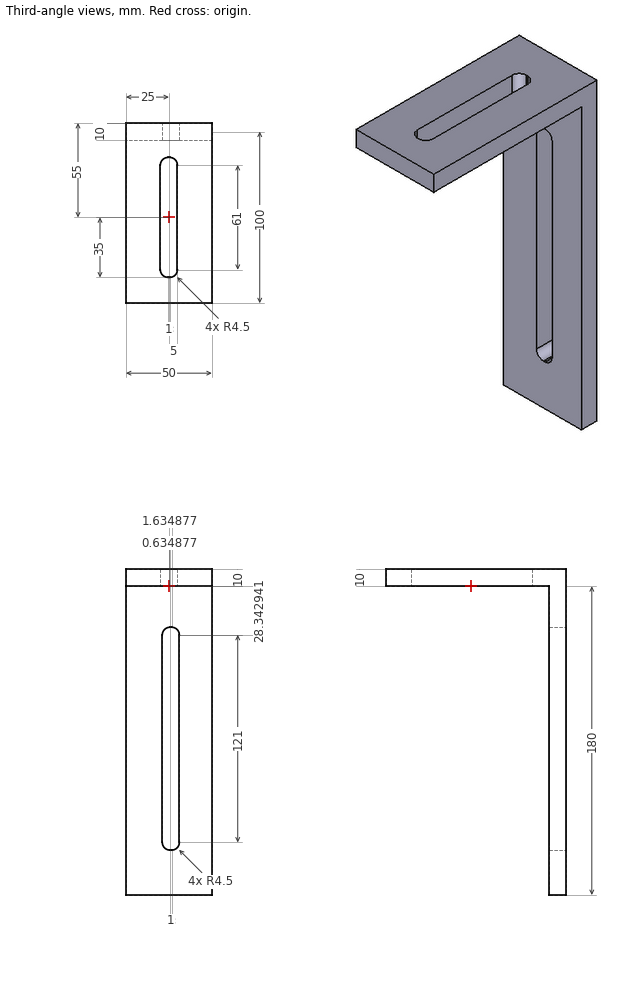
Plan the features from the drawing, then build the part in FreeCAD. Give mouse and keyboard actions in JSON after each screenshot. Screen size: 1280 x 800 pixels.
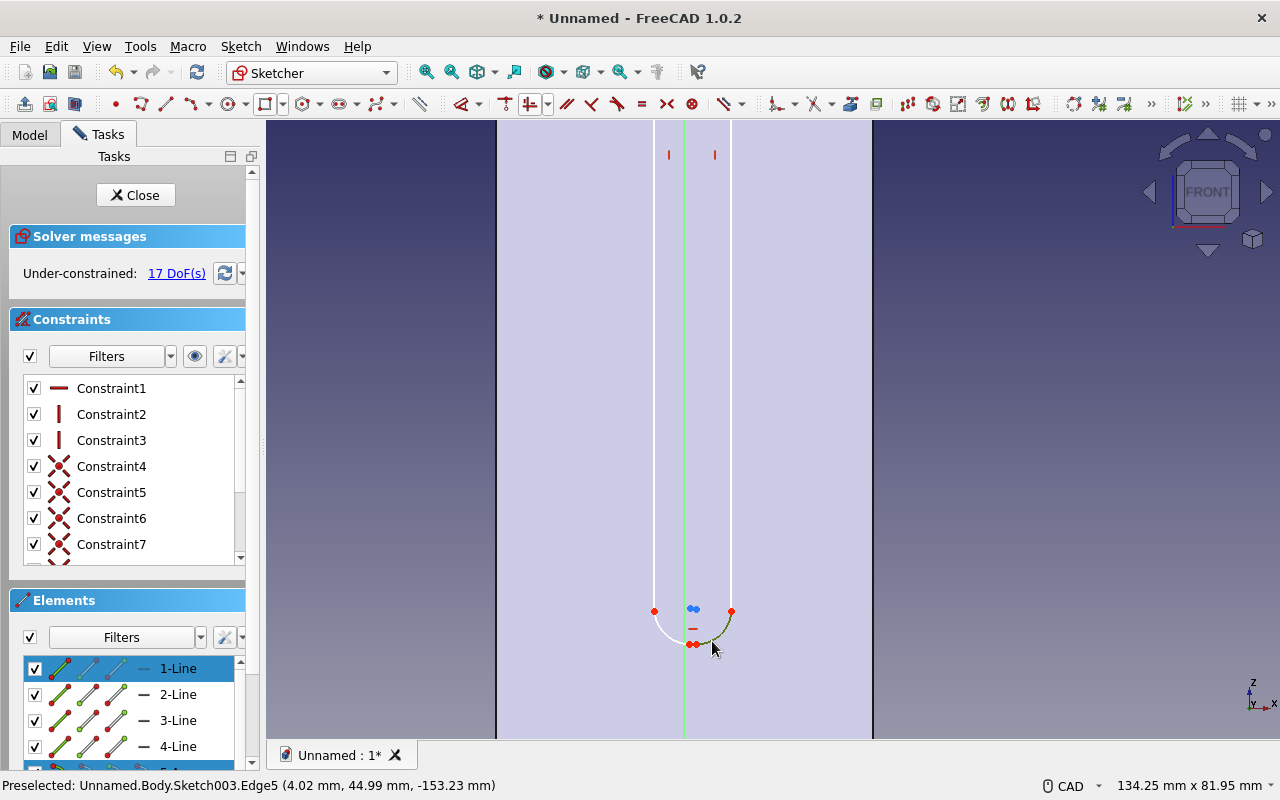
{"action": "left_click", "coordinate": [617, 104]}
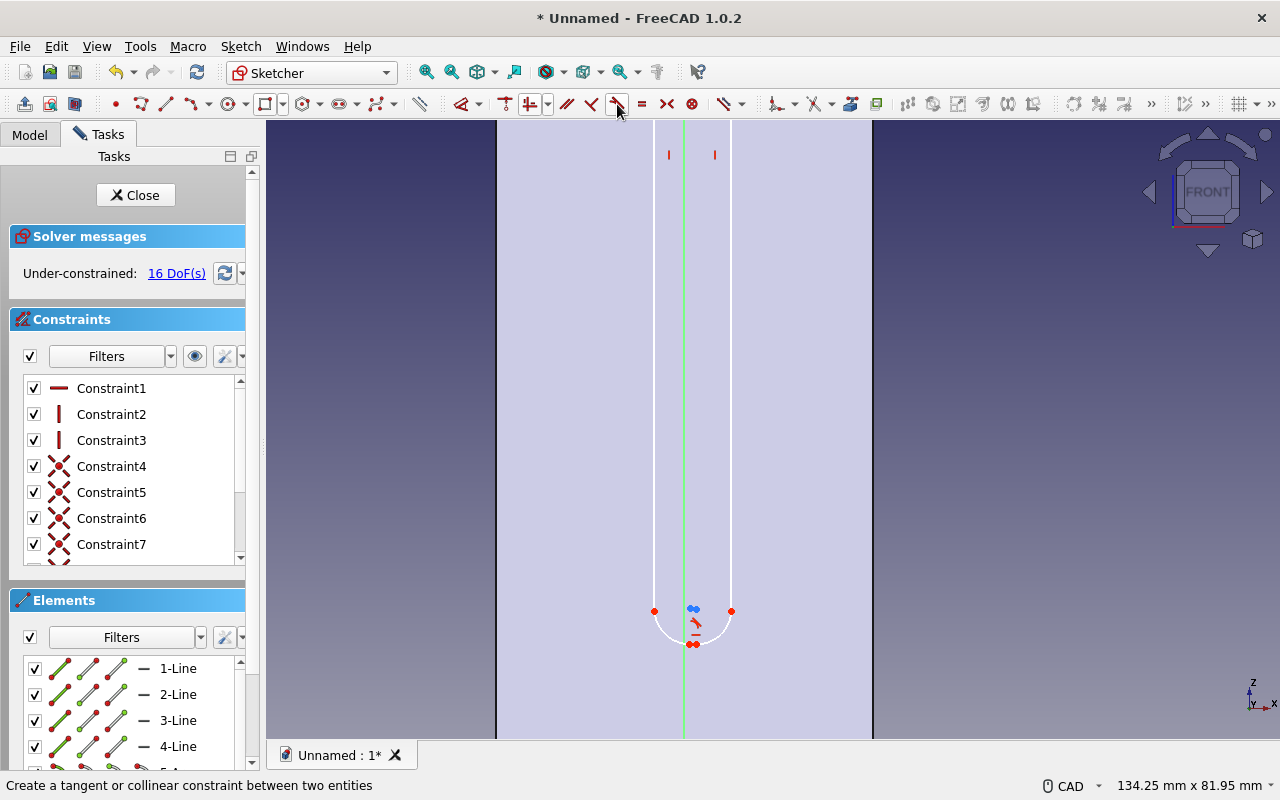
{"action": "scroll", "coordinate": [693, 644], "scroll_direction": "up", "scroll_amount": 7}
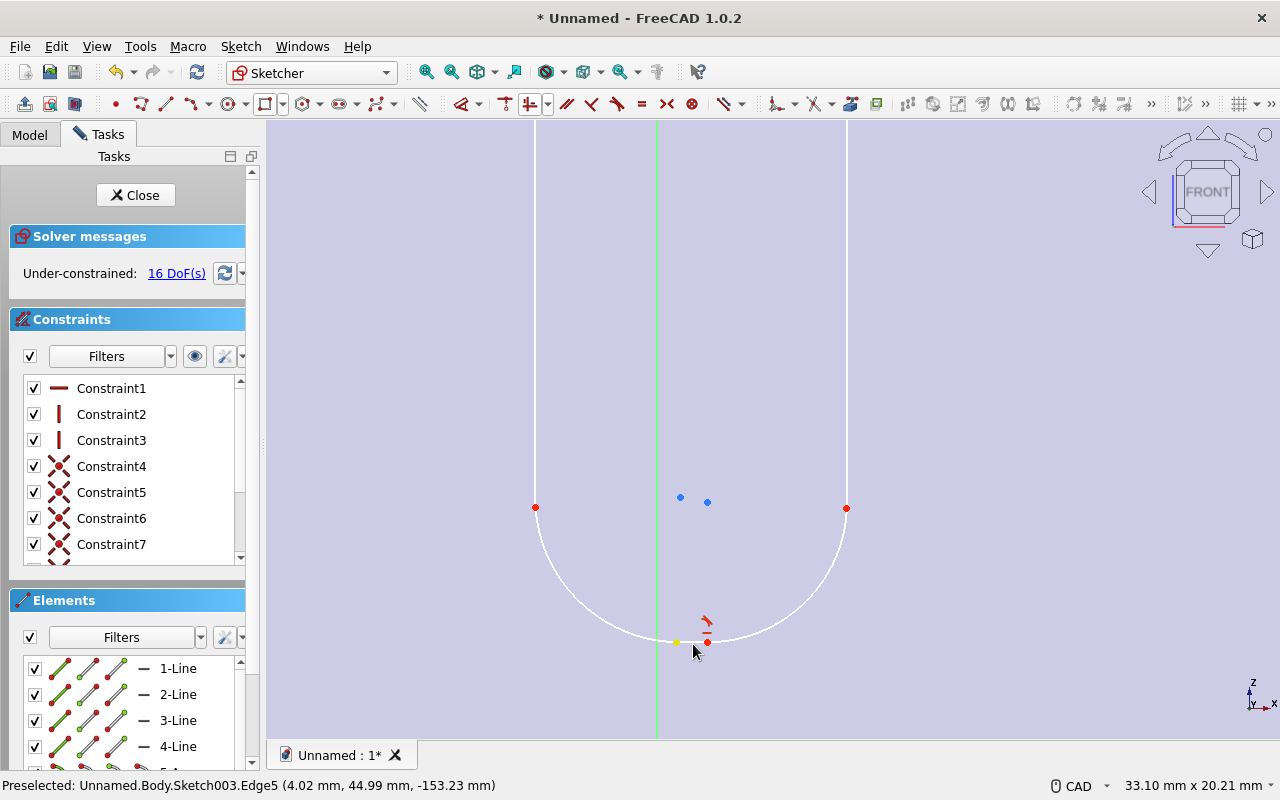
{"action": "left_click", "coordinate": [692, 642]}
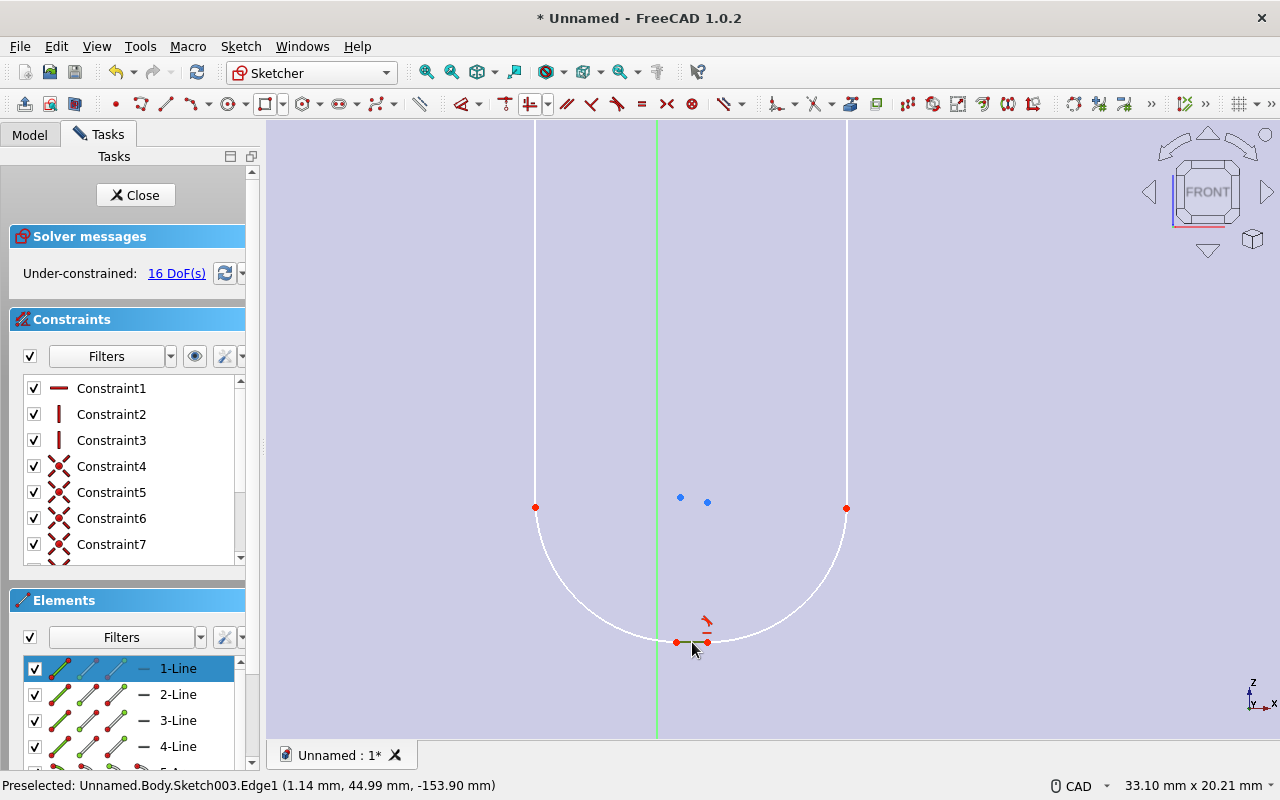
{"action": "scroll", "coordinate": [706, 644], "scroll_direction": "down", "scroll_amount": 12}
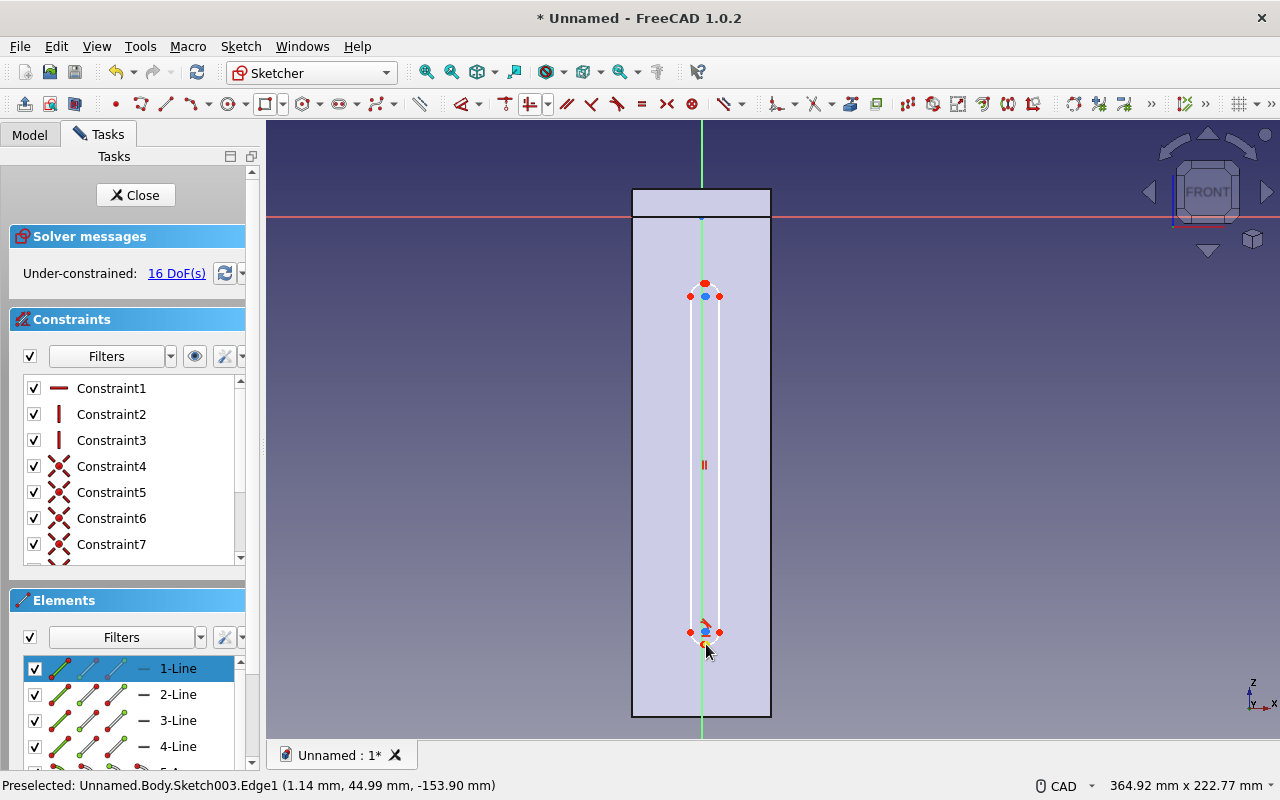
{"action": "scroll", "coordinate": [693, 638], "scroll_direction": "up", "scroll_amount": 5}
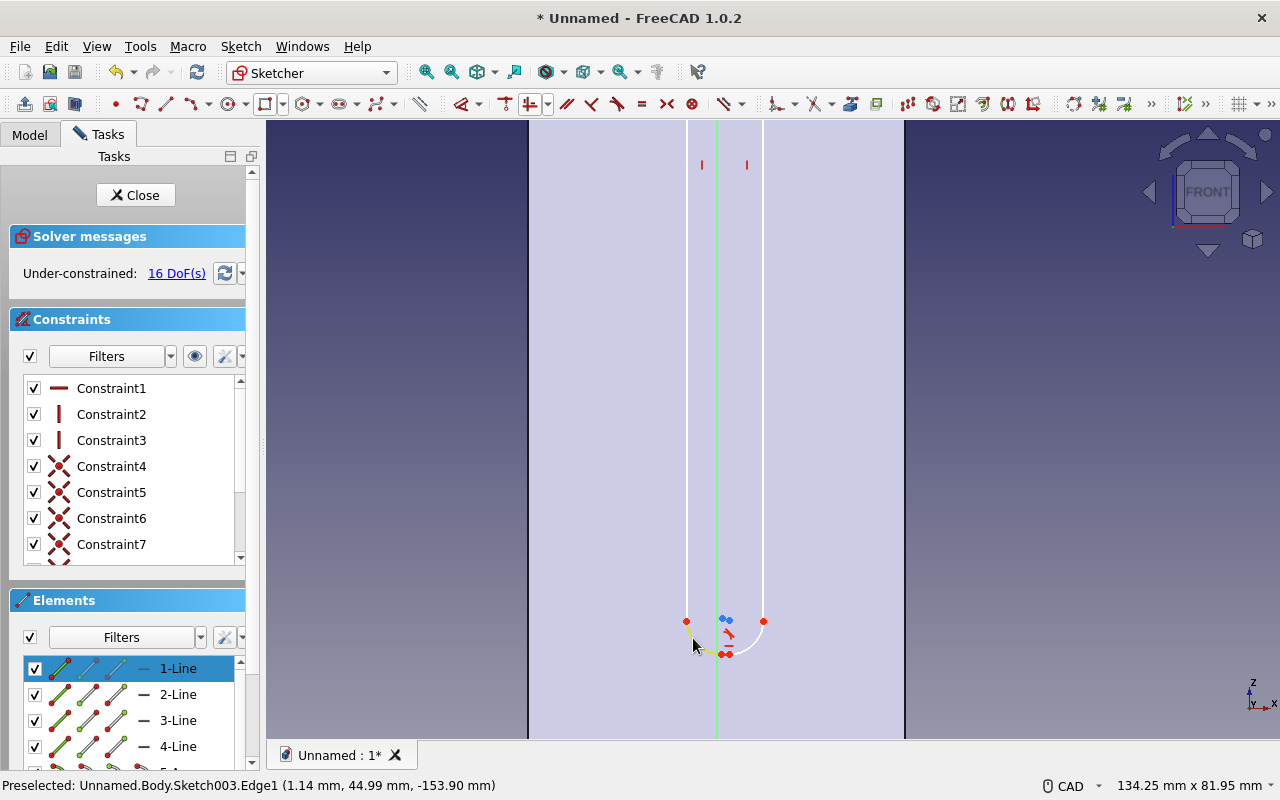
{"action": "left_click", "coordinate": [691, 636]}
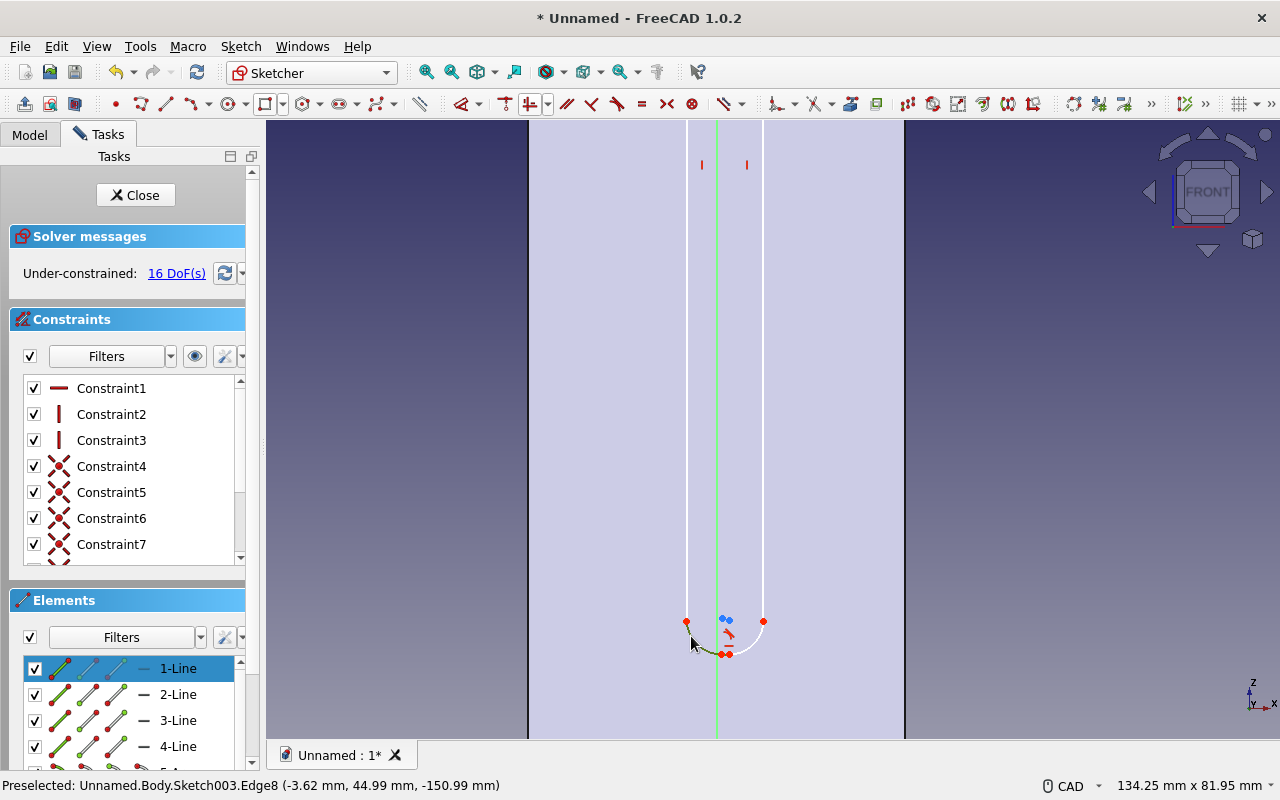
{"action": "left_click", "coordinate": [617, 104]}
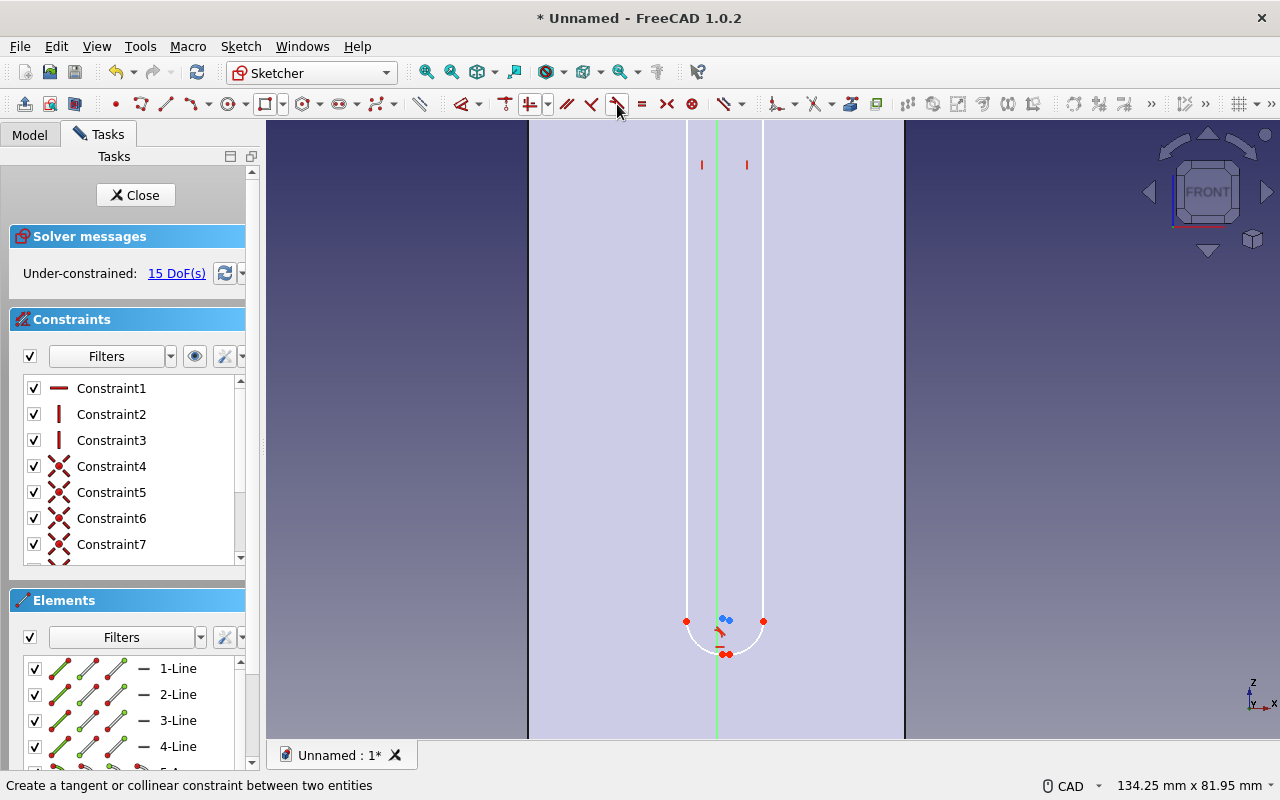
{"action": "left_click", "coordinate": [763, 348]}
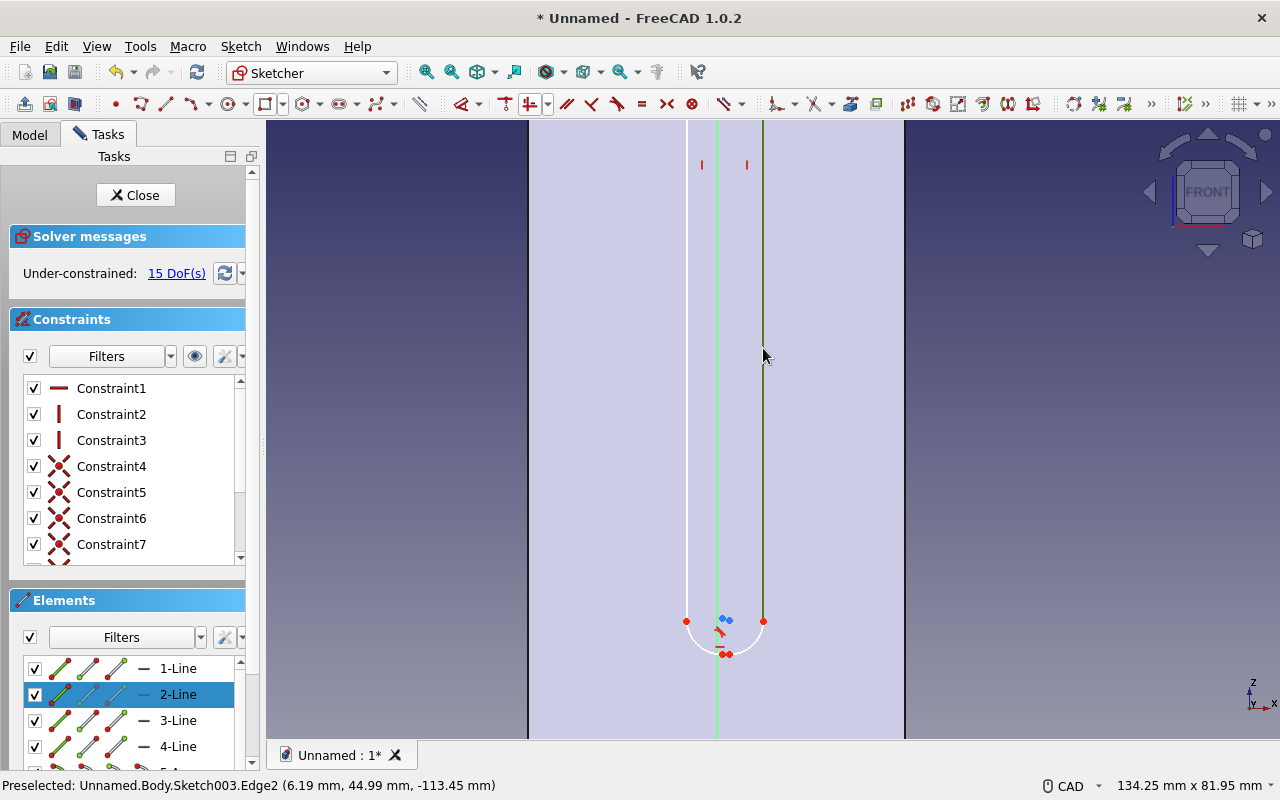
{"action": "left_click", "coordinate": [744, 651]}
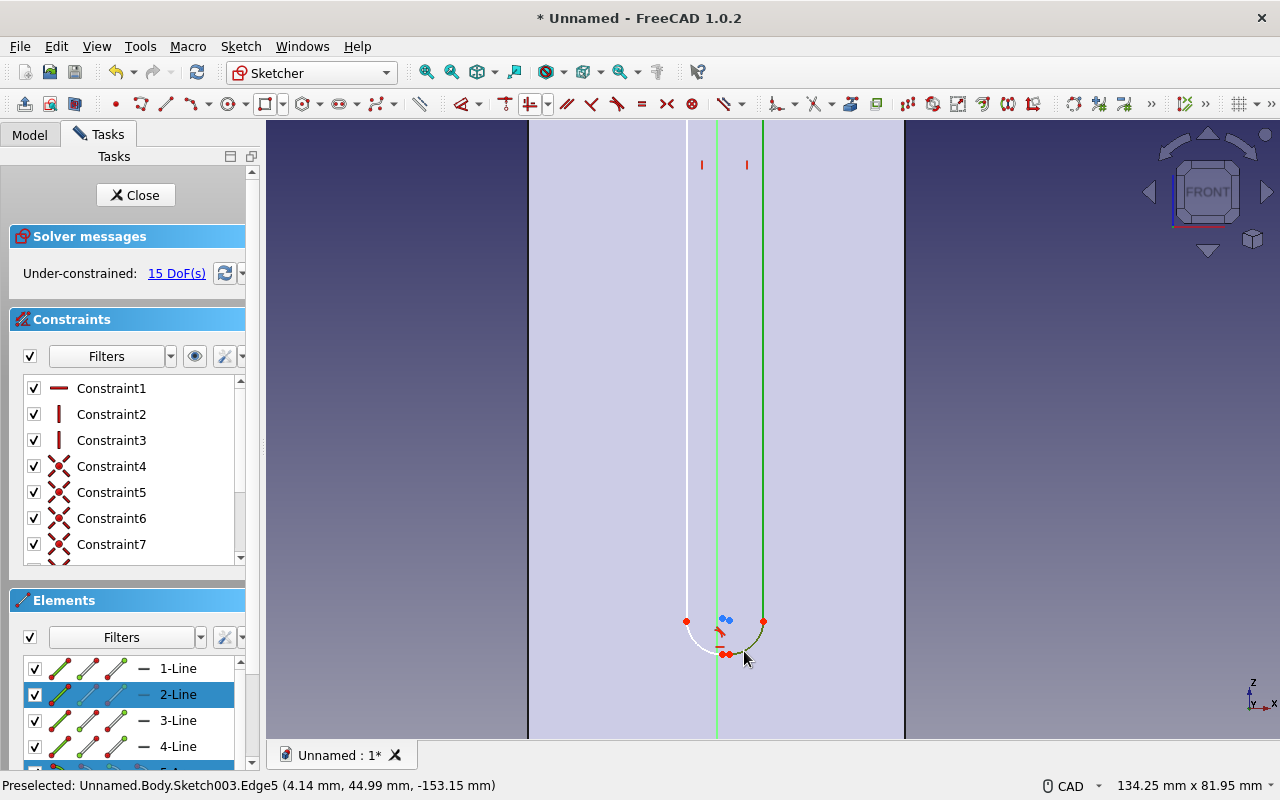
{"action": "left_click", "coordinate": [617, 104]}